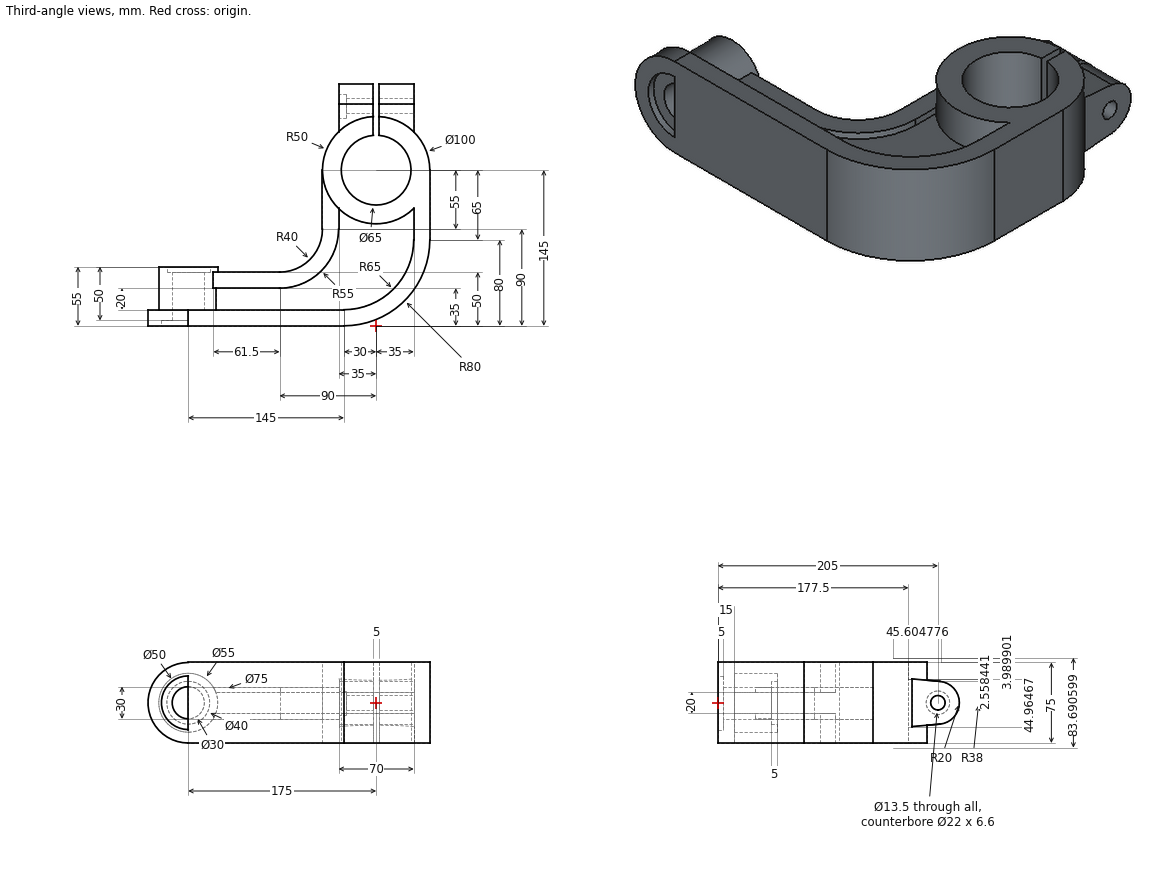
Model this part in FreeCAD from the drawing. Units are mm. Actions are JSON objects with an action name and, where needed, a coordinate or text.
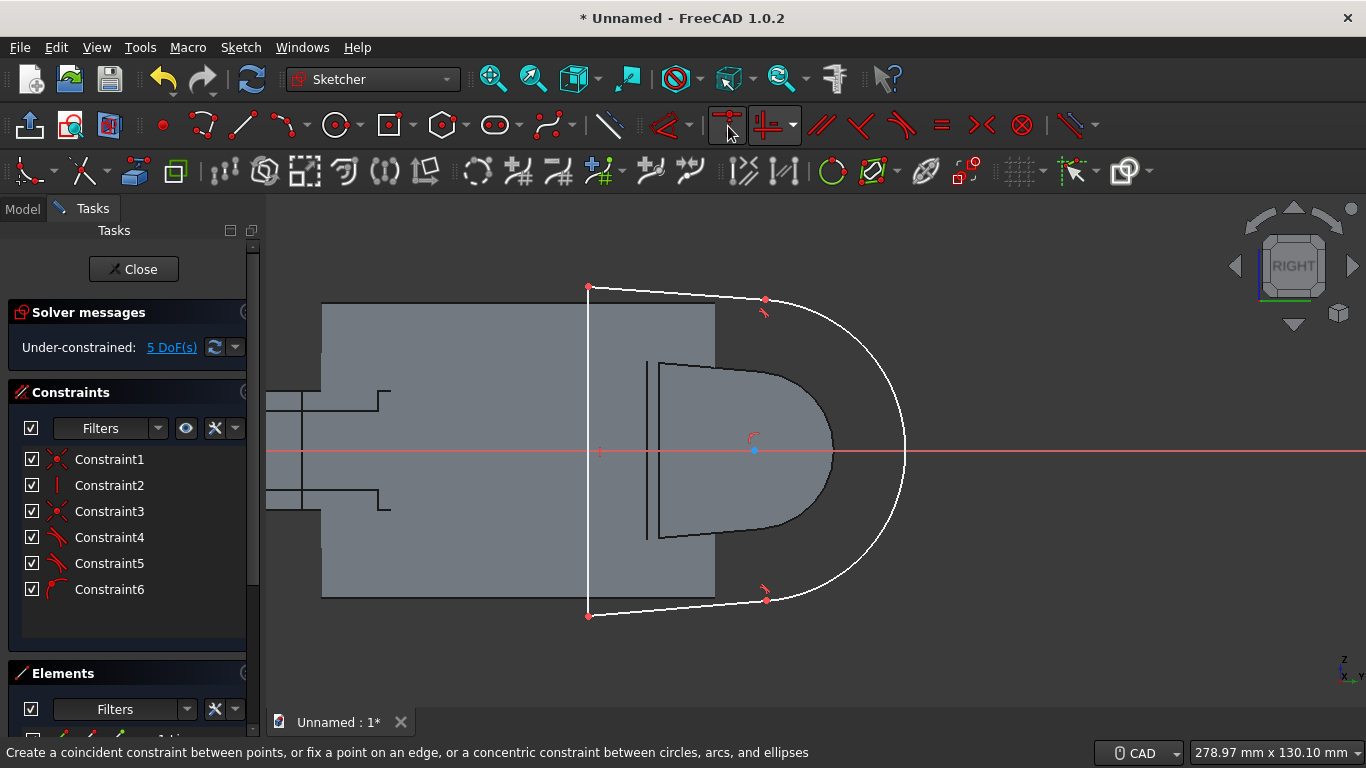
{"action": "key", "text": "d"}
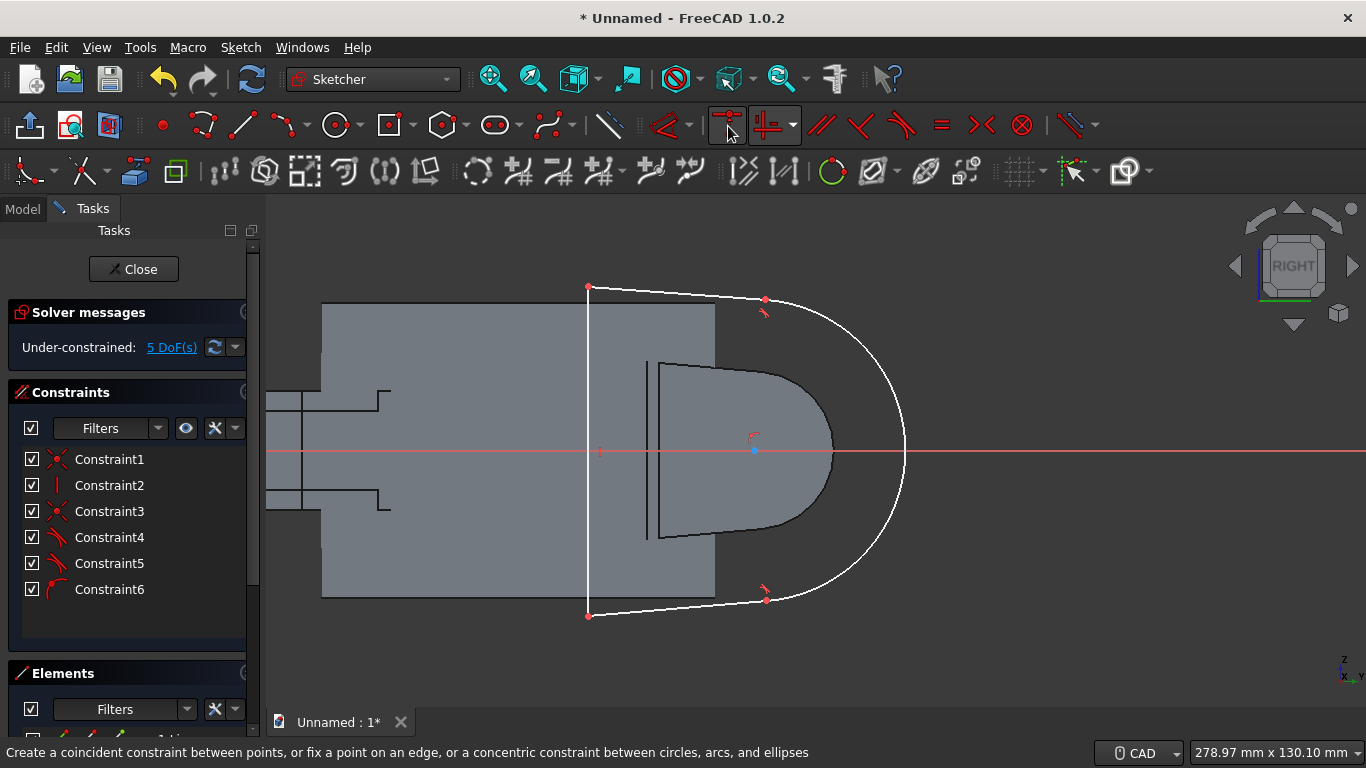
{"action": "left_click", "coordinate": [880, 535]}
{"action": "left_click", "coordinate": [907, 553]}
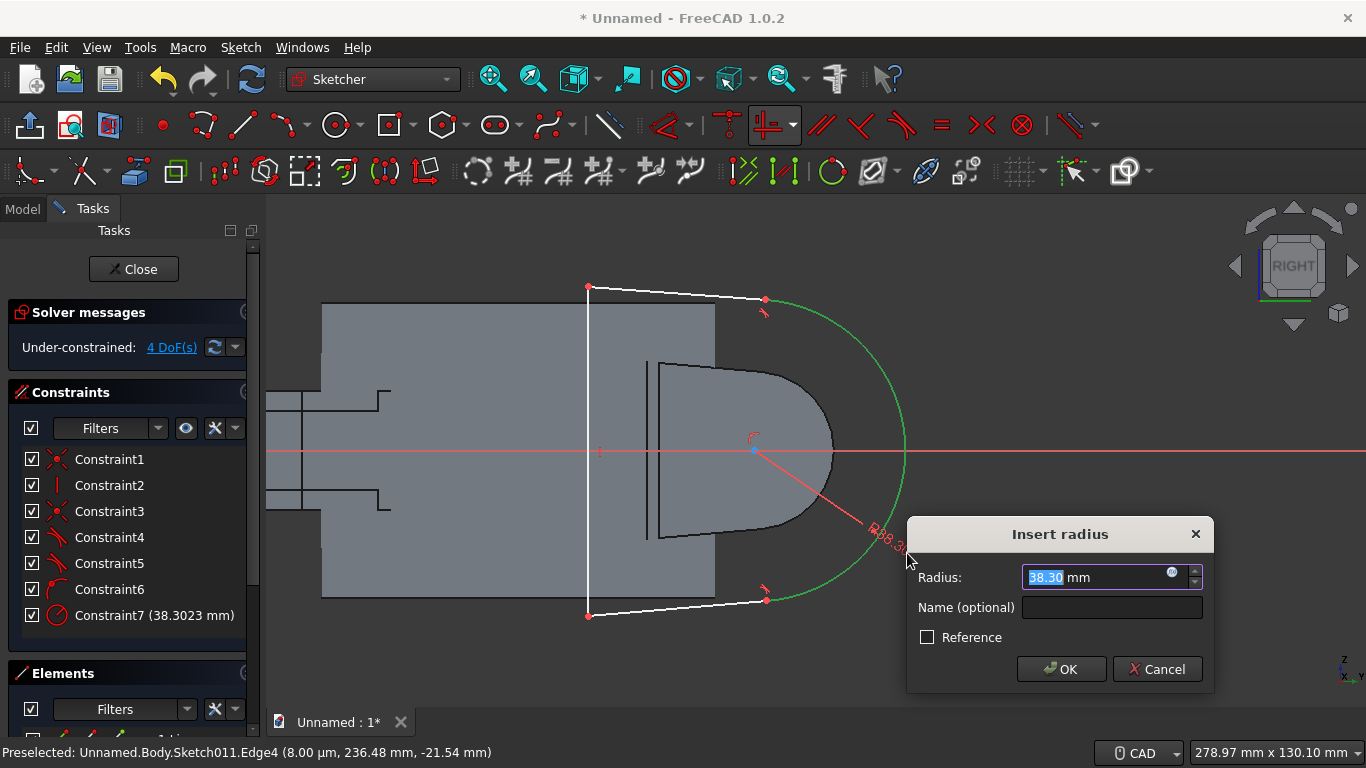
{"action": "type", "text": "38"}
{"action": "key", "text": "Return"}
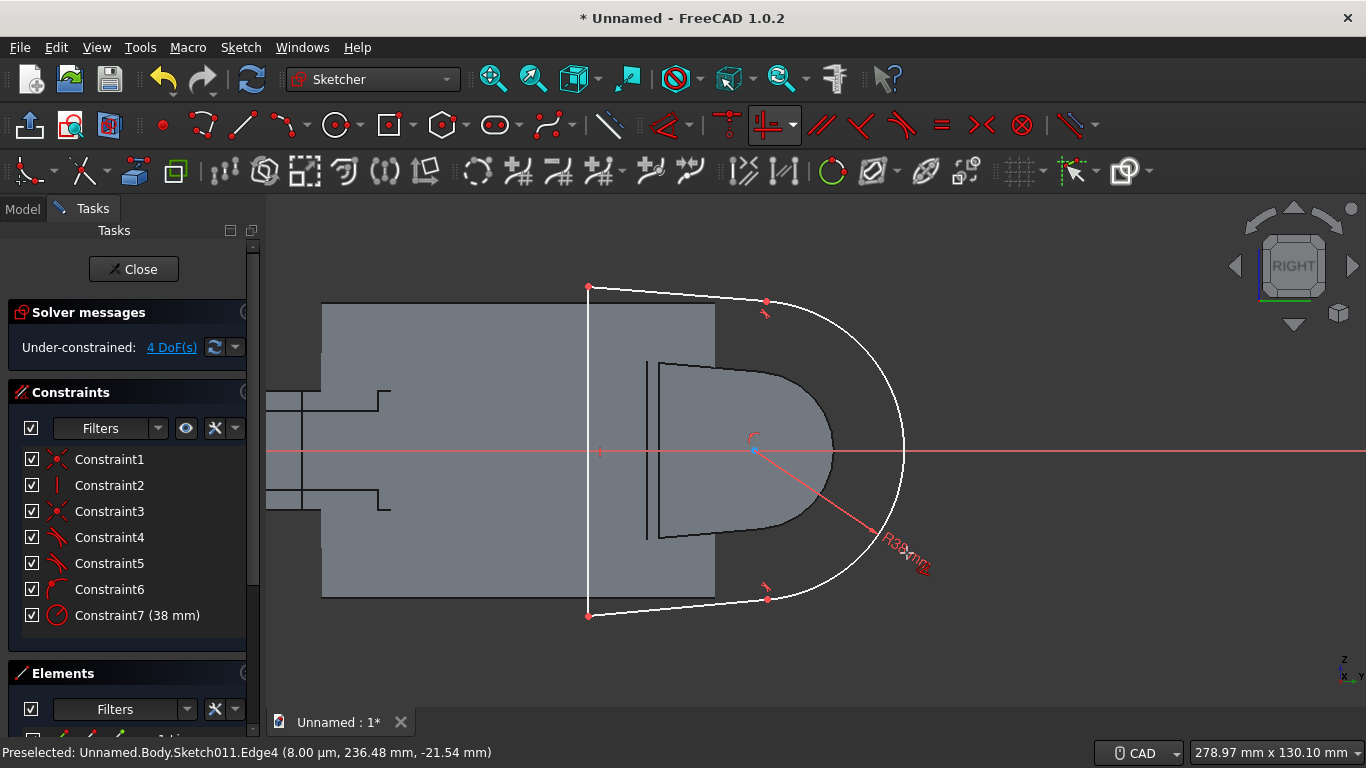
{"action": "left_click", "coordinate": [754, 450]}
{"action": "left_click", "coordinate": [524, 484]}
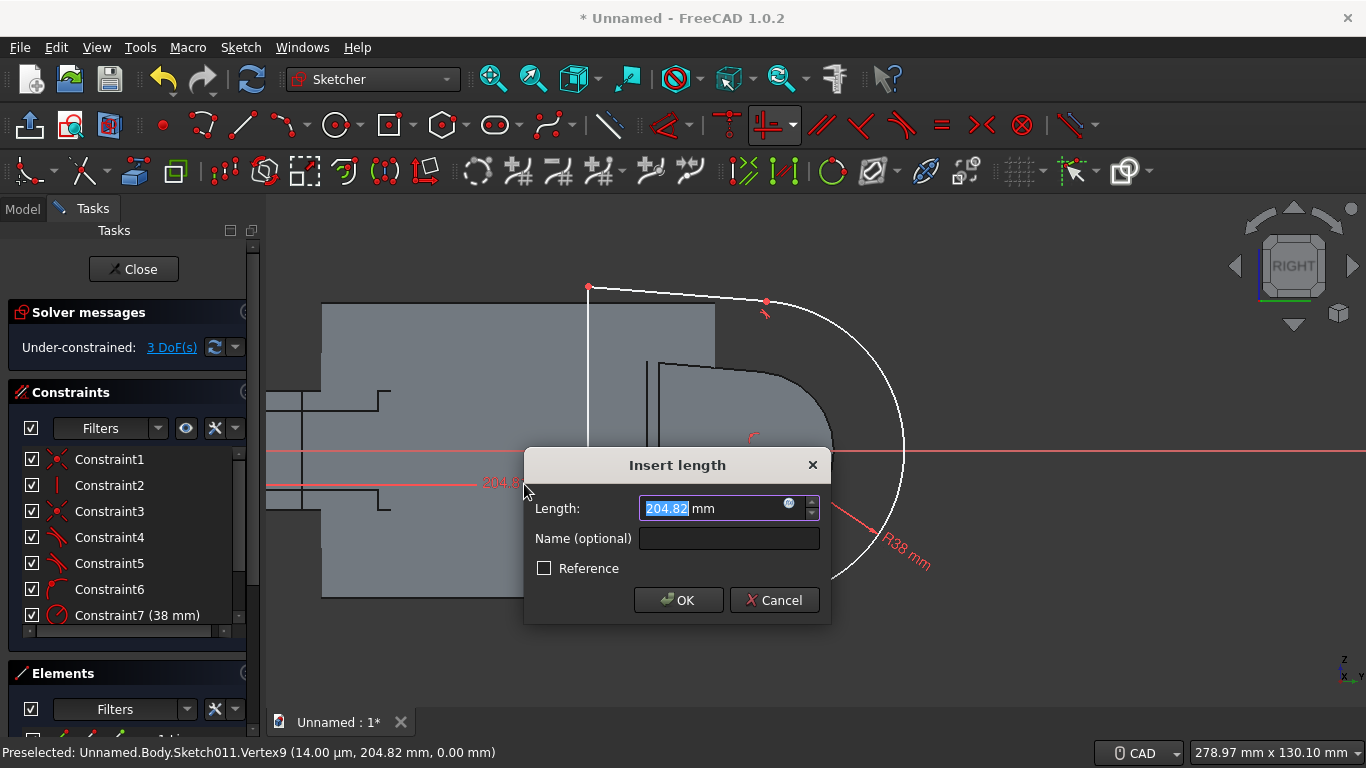
{"action": "type", "text": "205"}
{"action": "key", "text": "Return"}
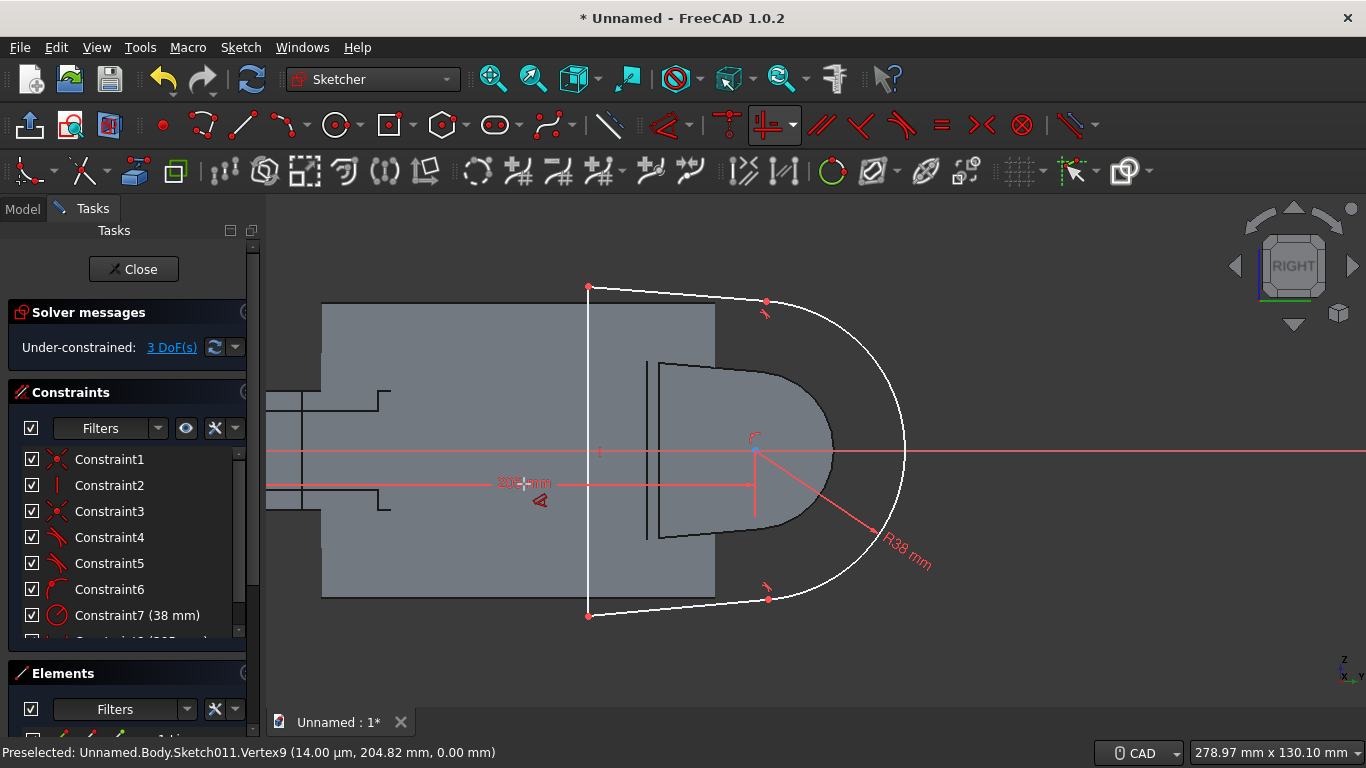
{"action": "left_click", "coordinate": [588, 386]}
{"action": "left_click", "coordinate": [554, 376]}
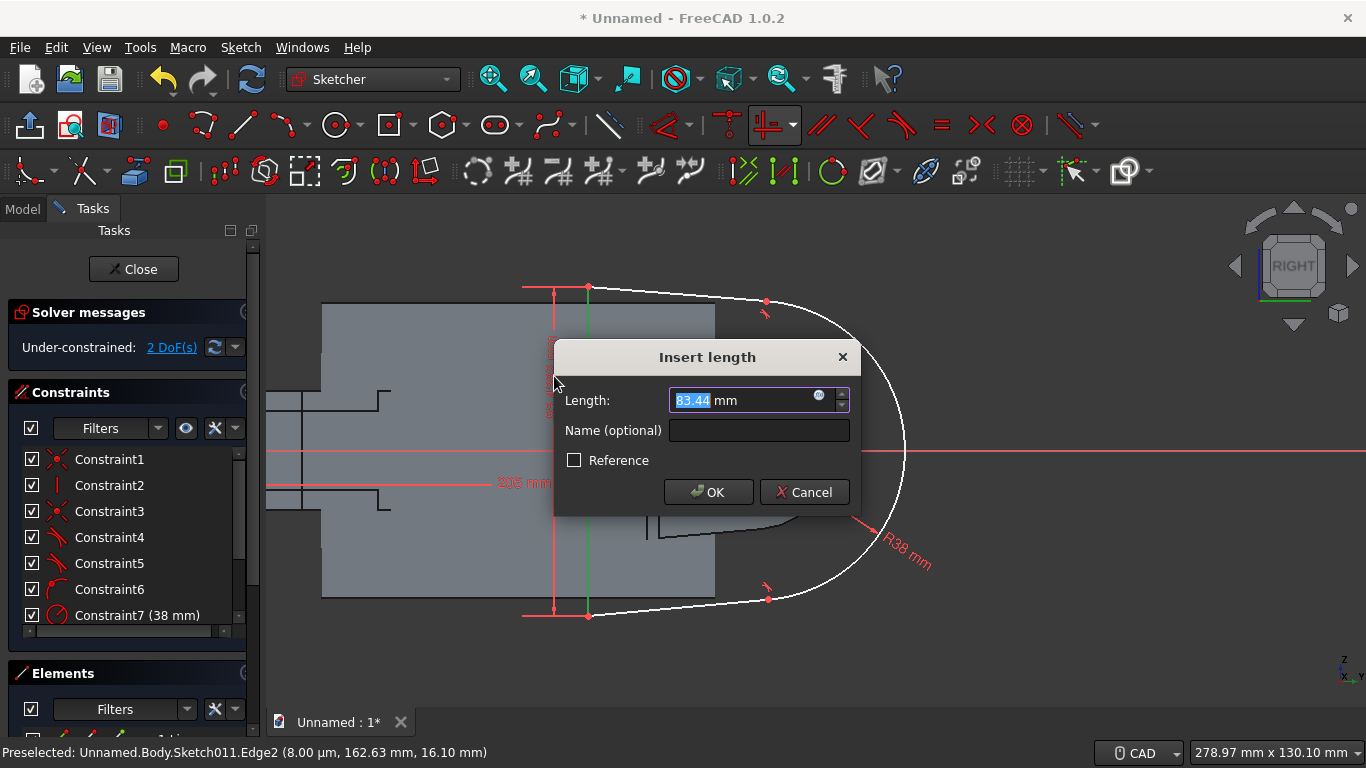
{"action": "type", "text": "83.690599"}
{"action": "key", "text": "Return"}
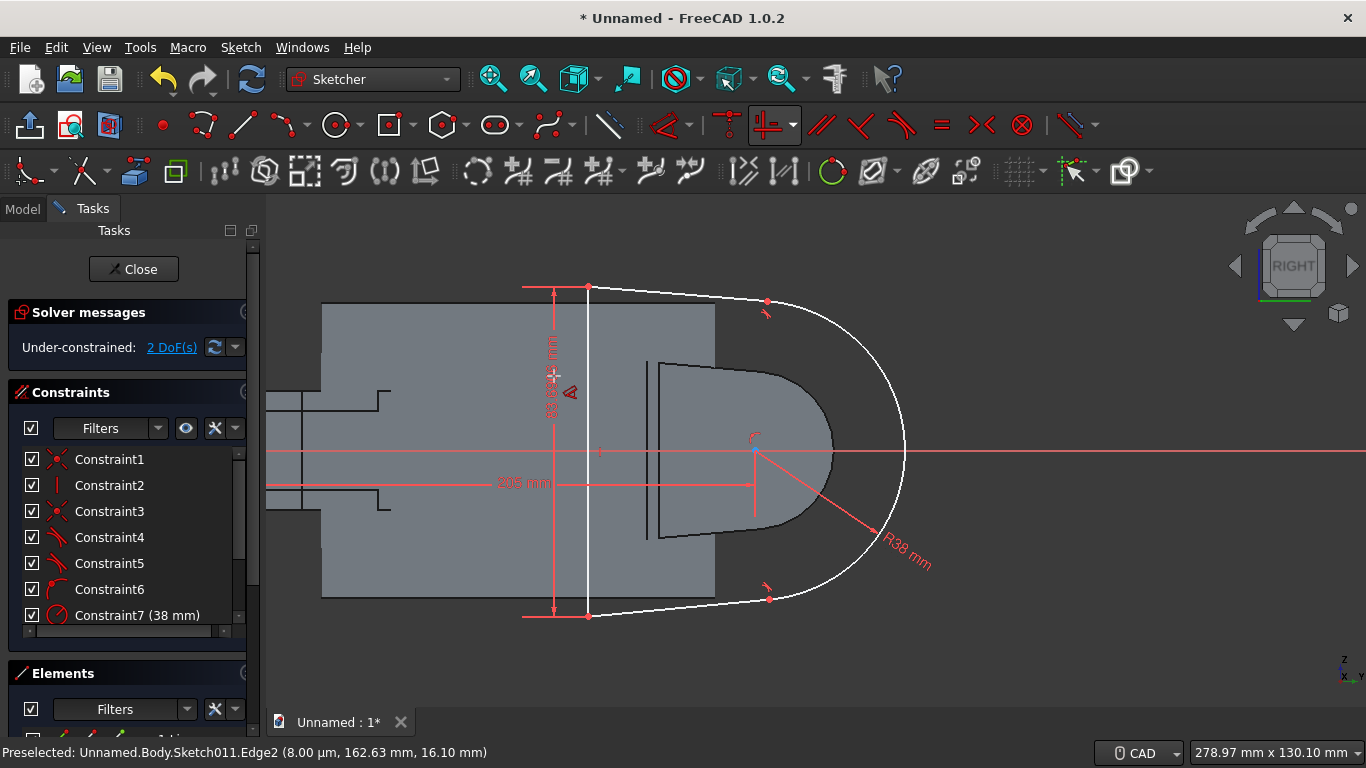
{"action": "scroll", "coordinate": [713, 297], "scroll_direction": "up", "scroll_amount": 5}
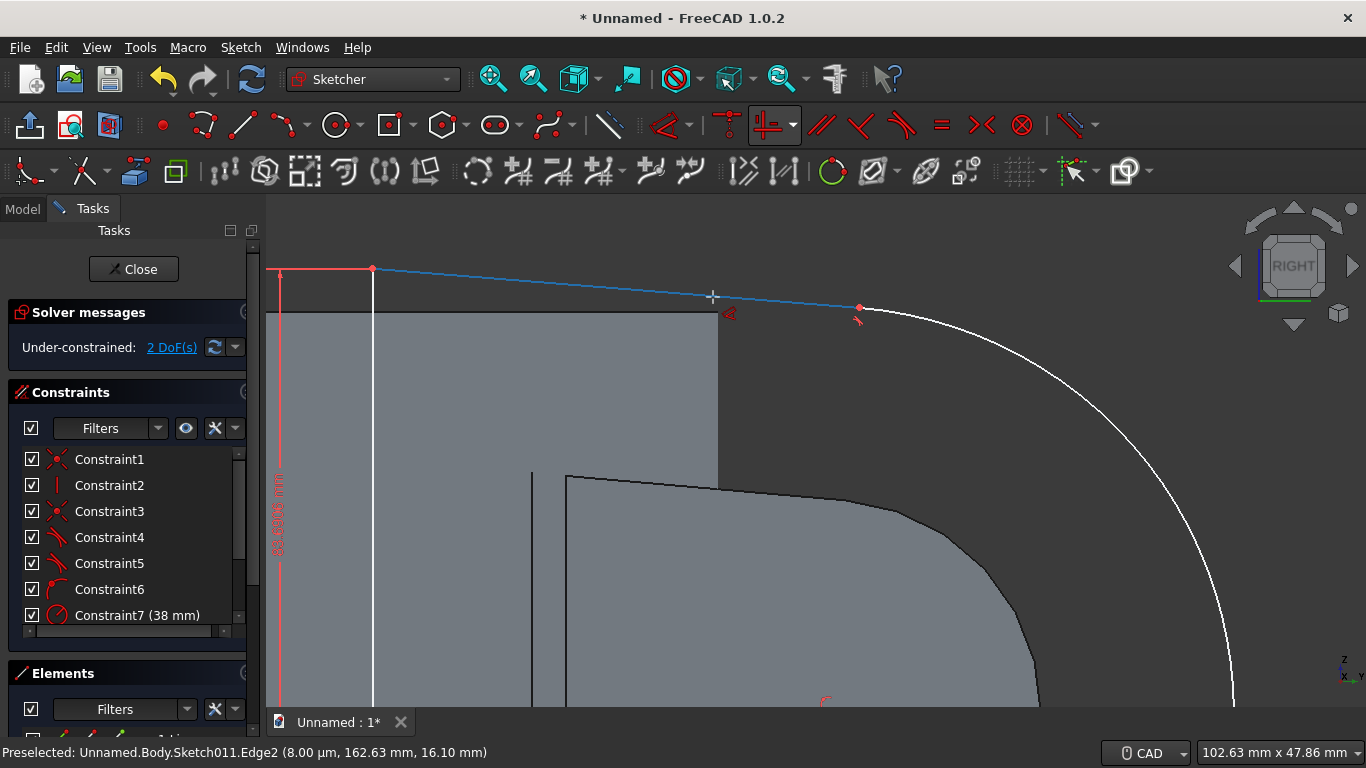
{"action": "left_click", "coordinate": [713, 296]}
{"action": "left_click", "coordinate": [339, 288]}